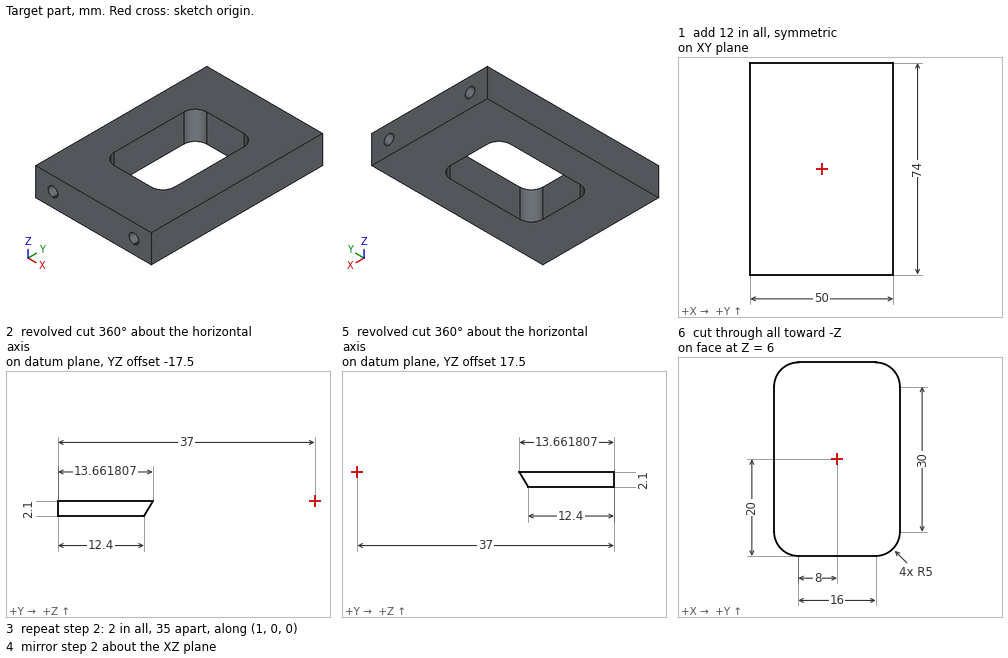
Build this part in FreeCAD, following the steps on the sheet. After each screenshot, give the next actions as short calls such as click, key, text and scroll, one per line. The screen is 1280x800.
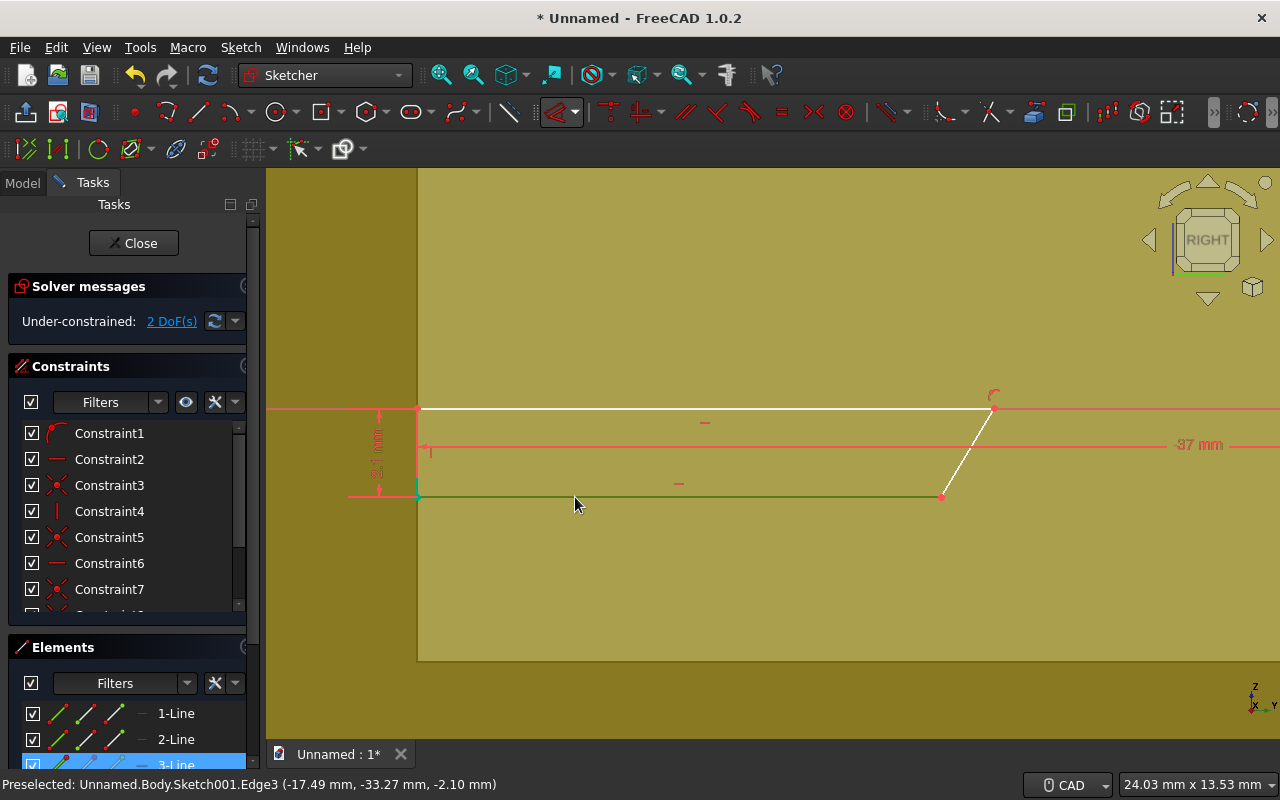
click(578, 112)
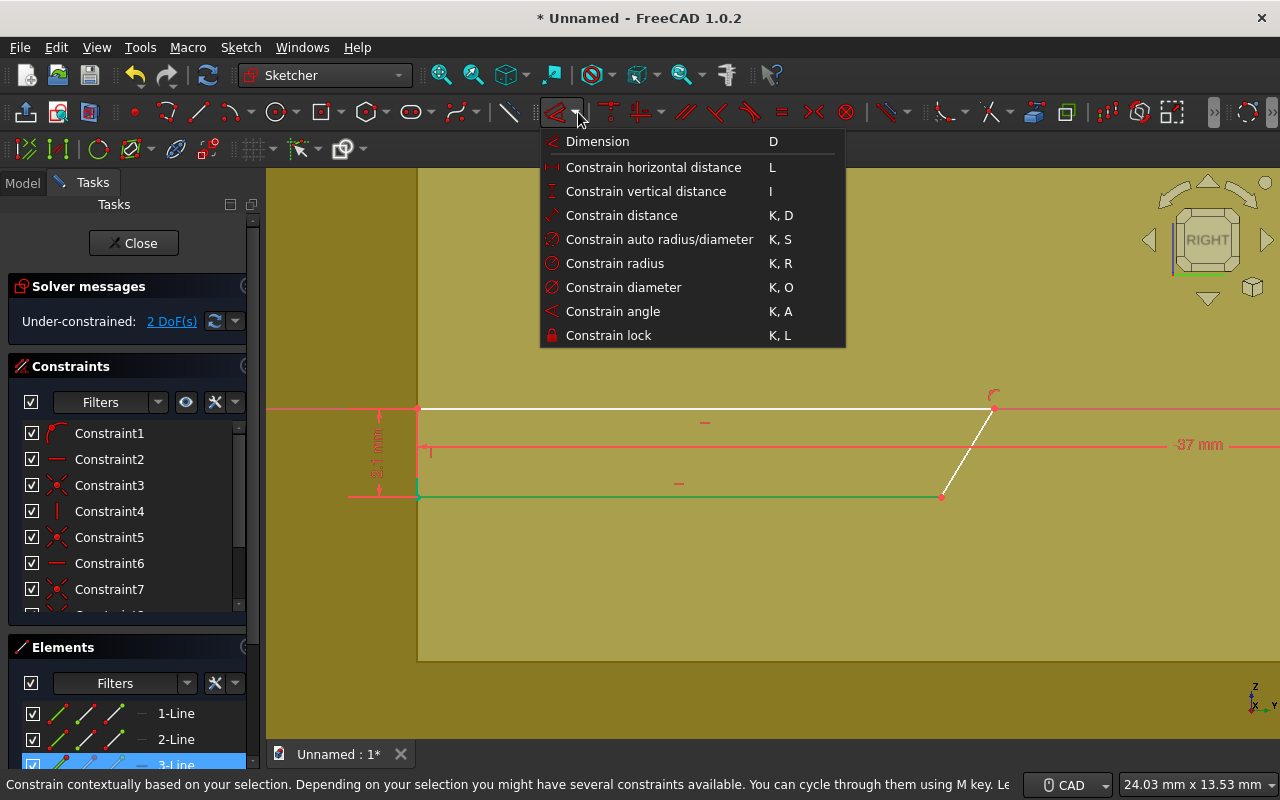
click(693, 167)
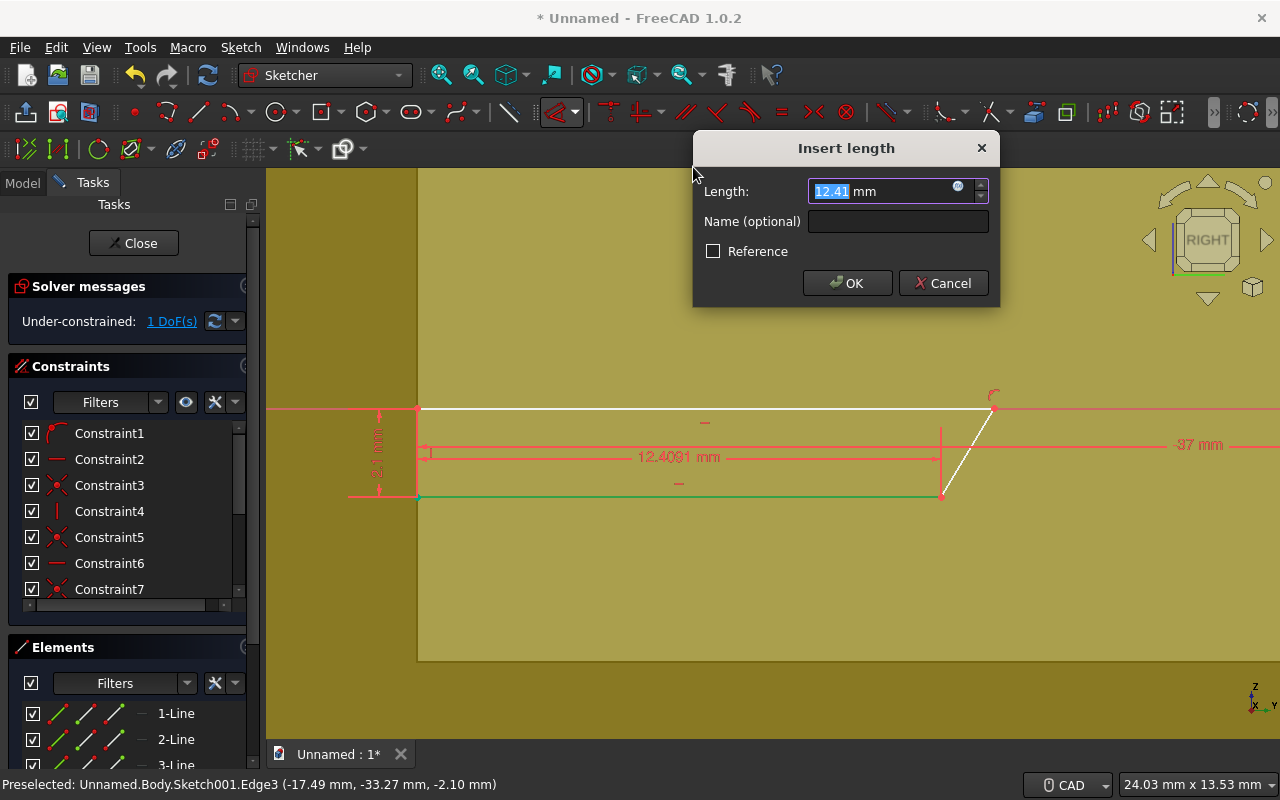
text(12.4)
key(Return)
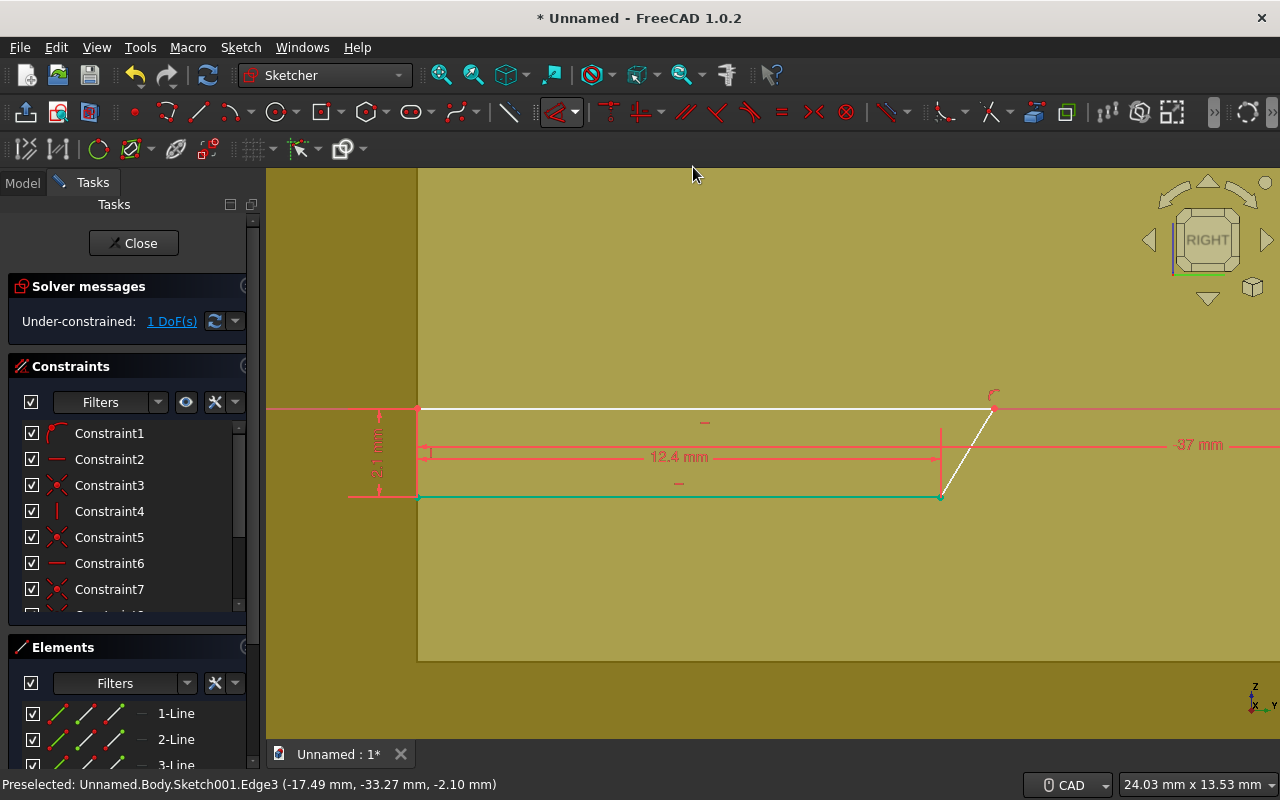
click(821, 409)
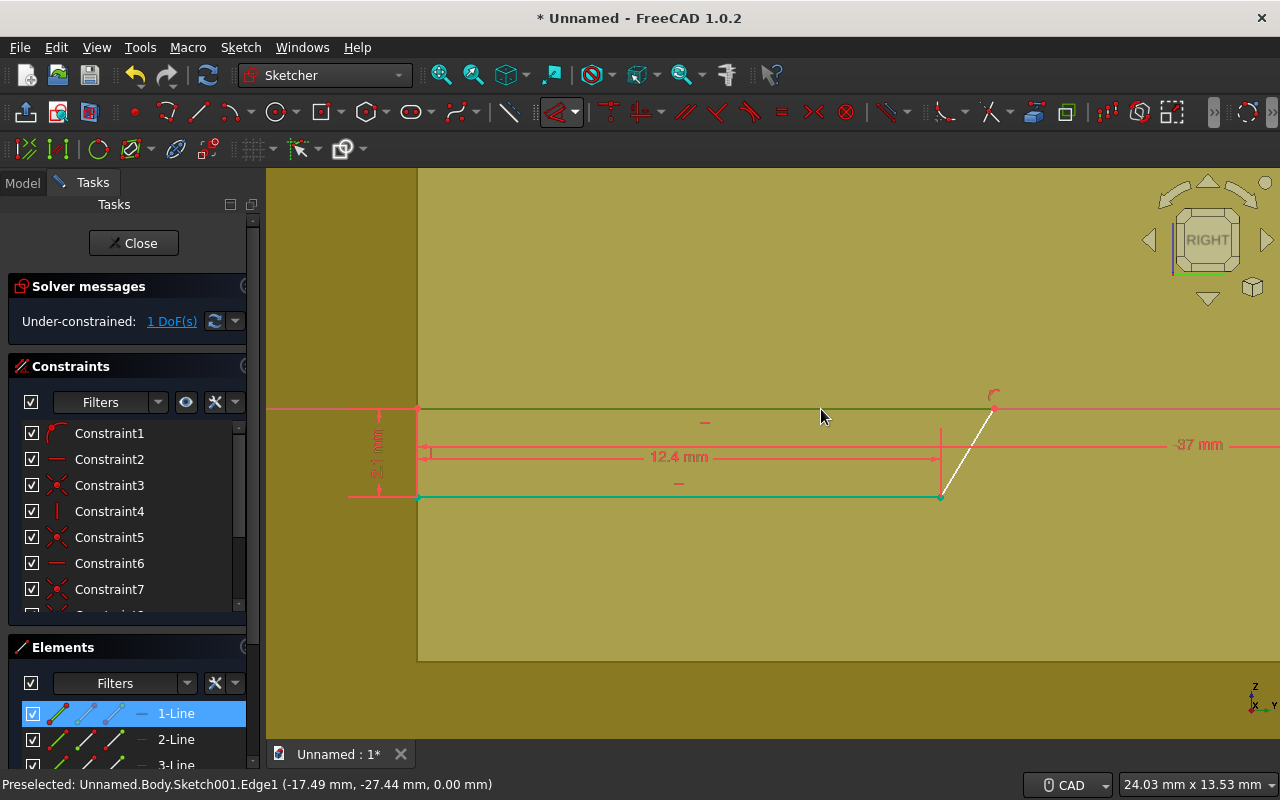
key(l)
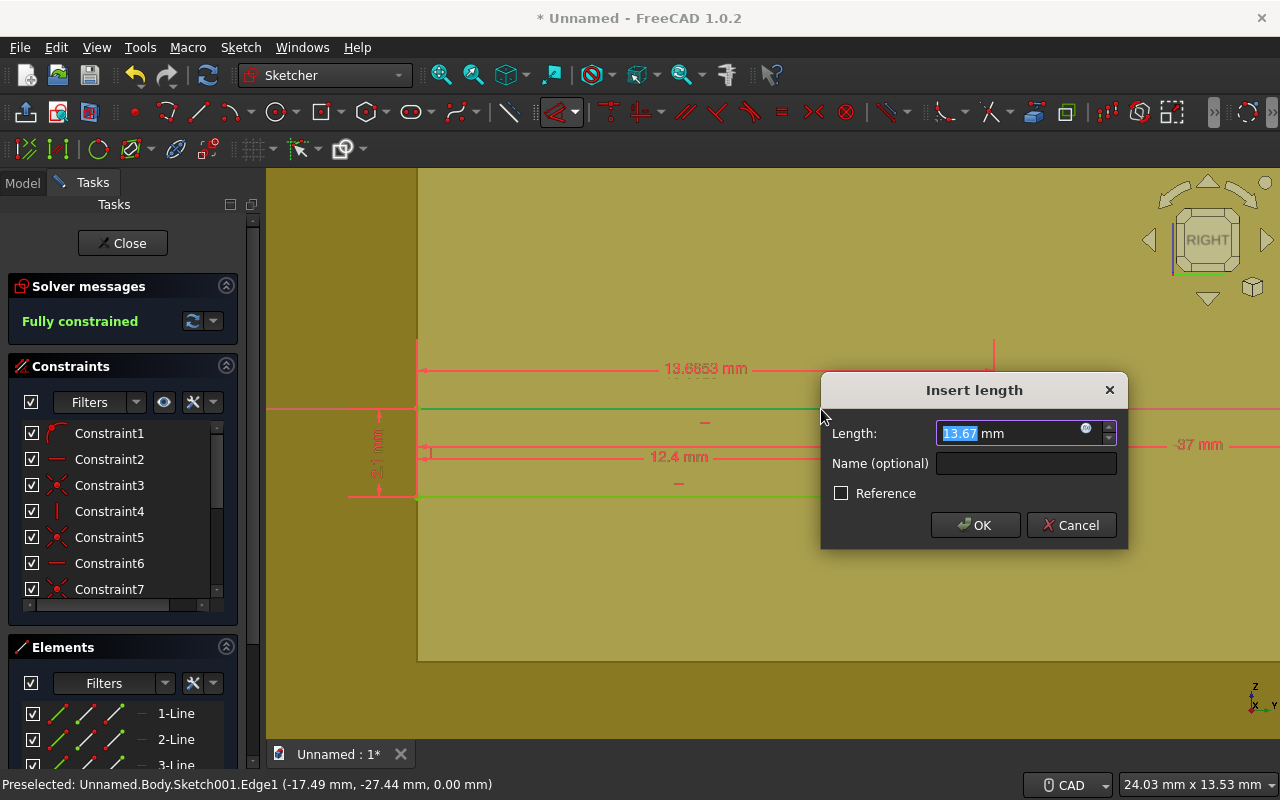
text(13.661807)
key(Return)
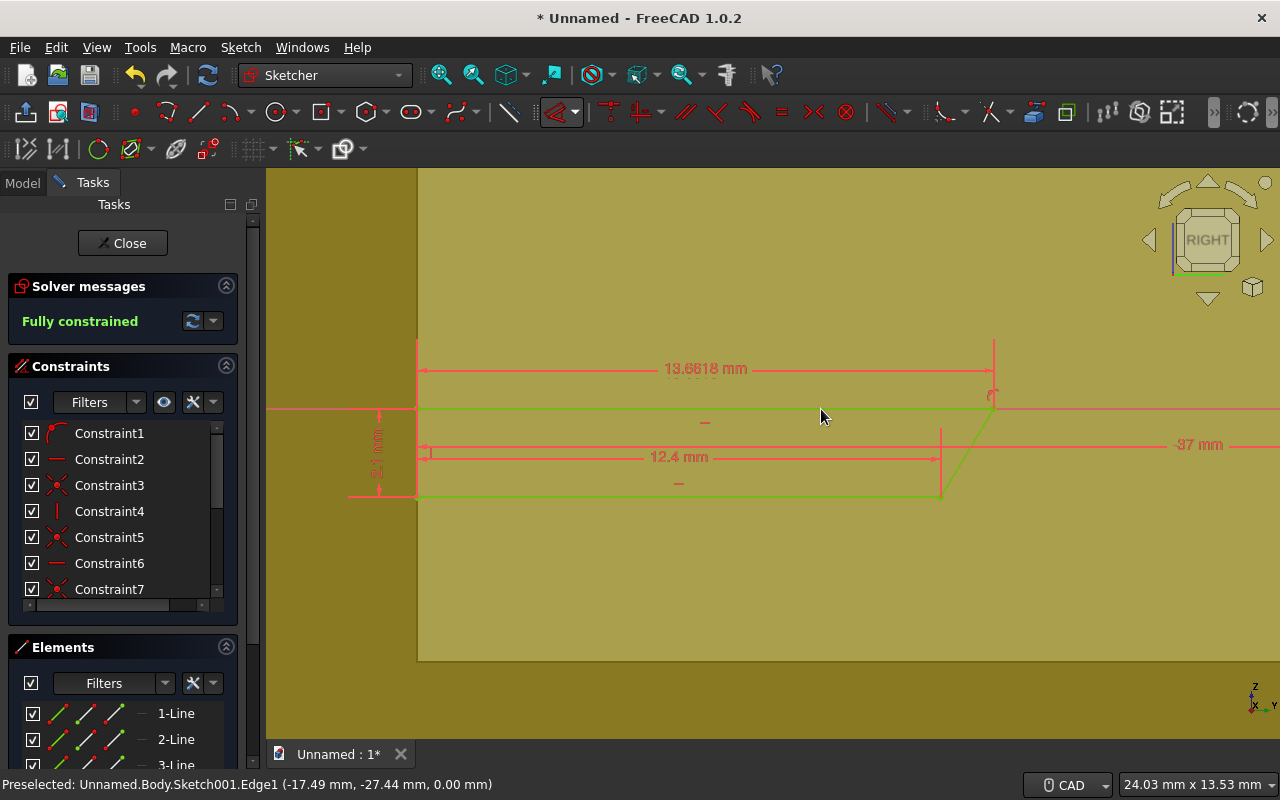
click(123, 243)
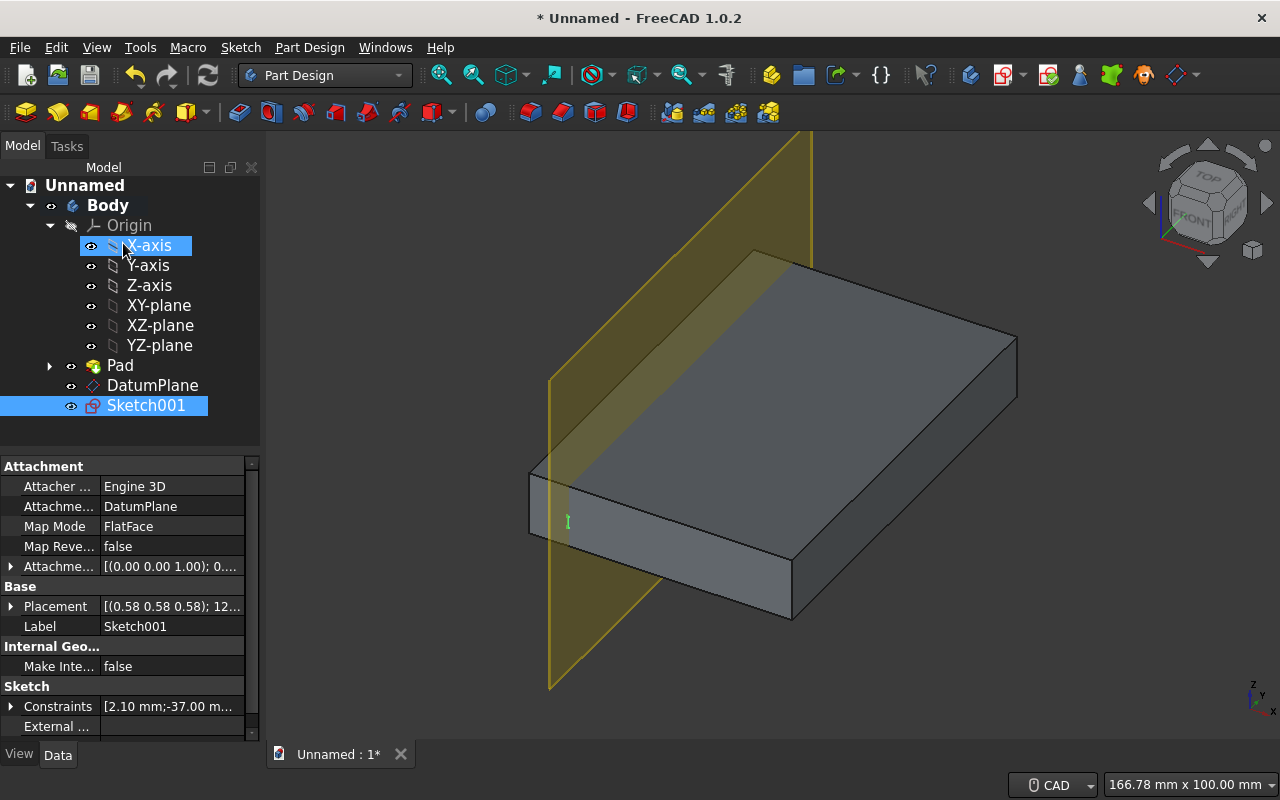
click(304, 112)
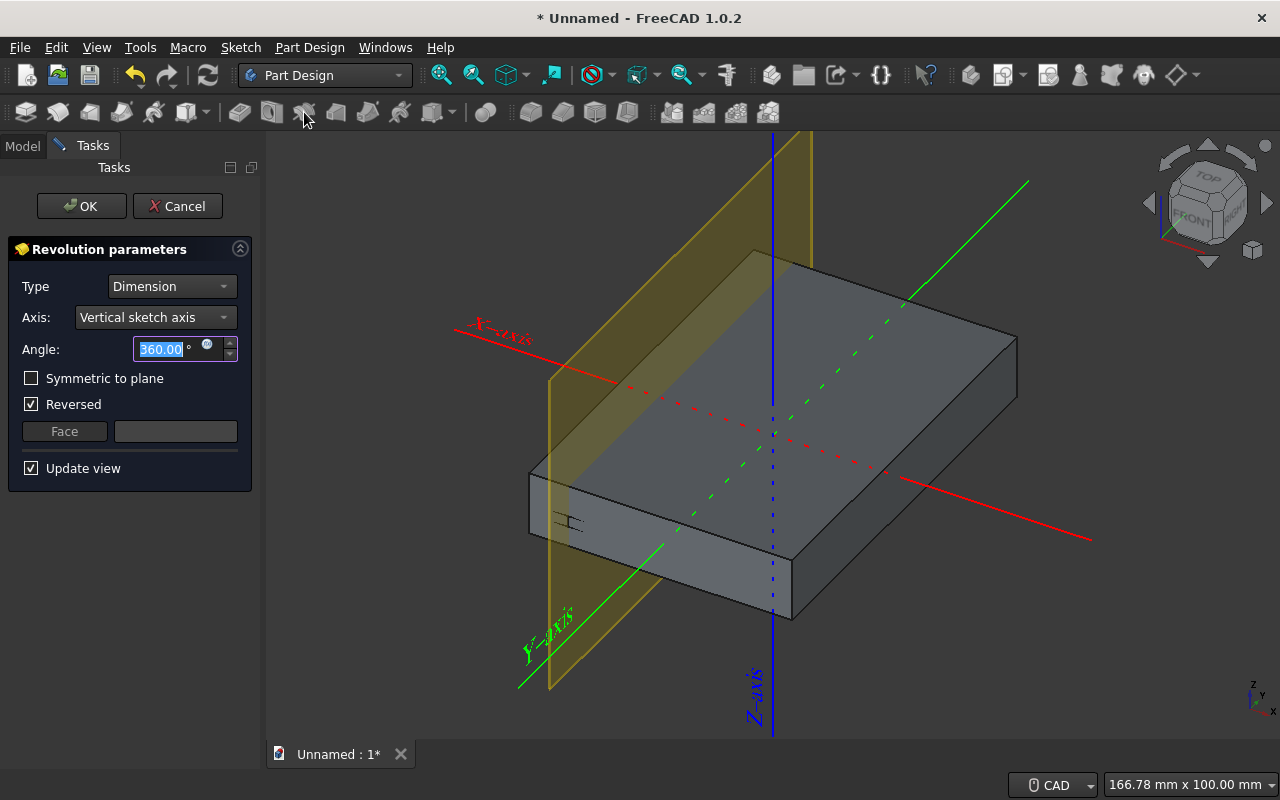
click(156, 318)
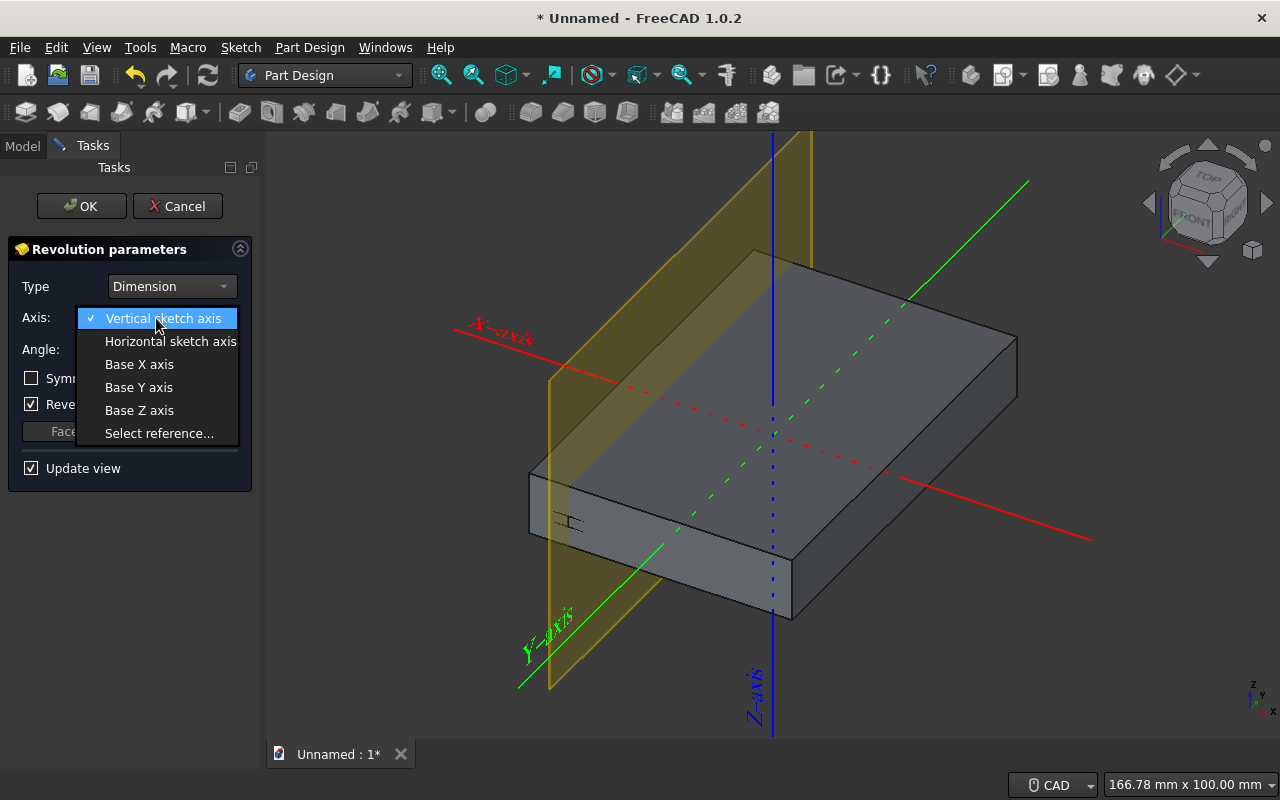
click(156, 342)